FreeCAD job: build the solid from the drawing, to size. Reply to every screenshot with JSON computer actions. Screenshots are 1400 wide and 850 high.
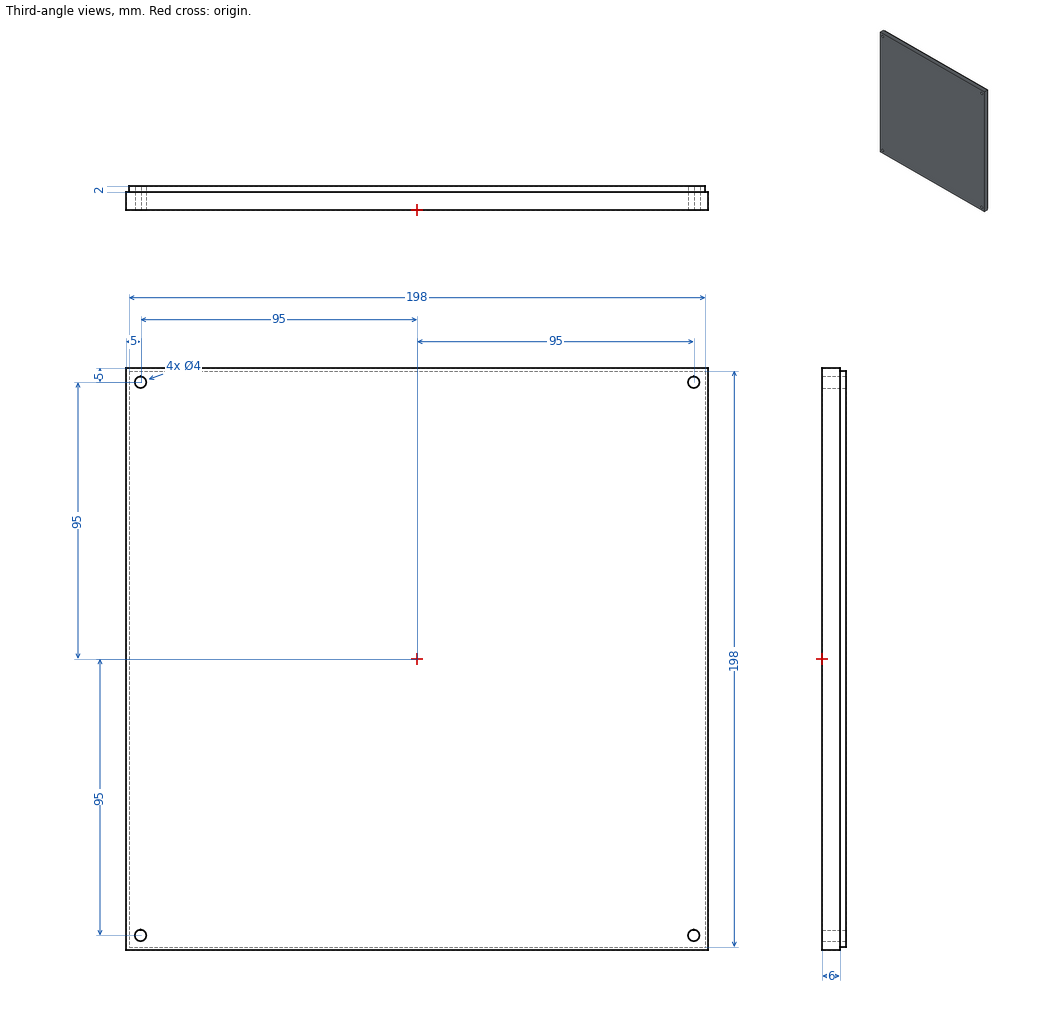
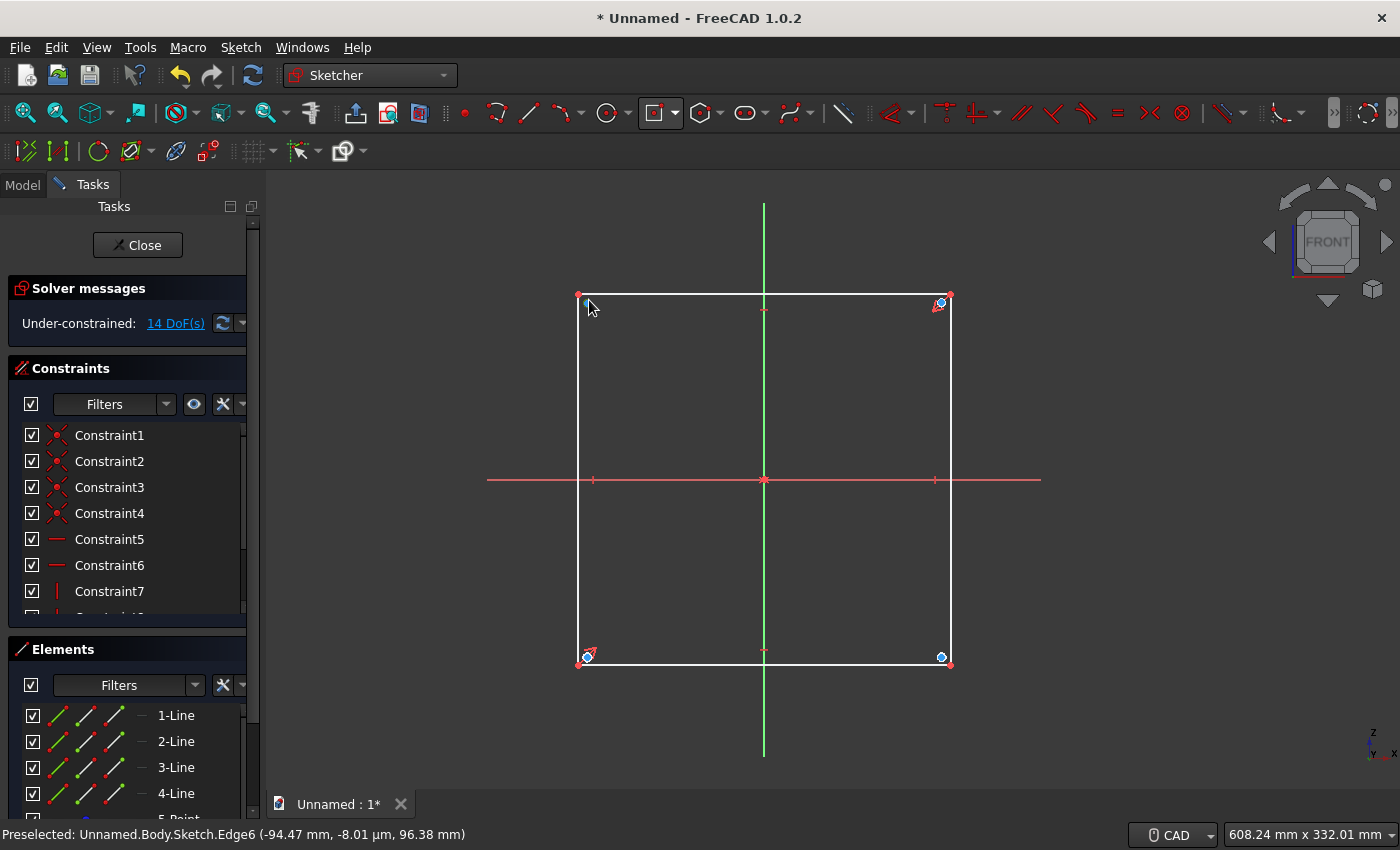
{"action": "scroll", "coordinate": [944, 300], "scroll_direction": "up", "scroll_amount": 7}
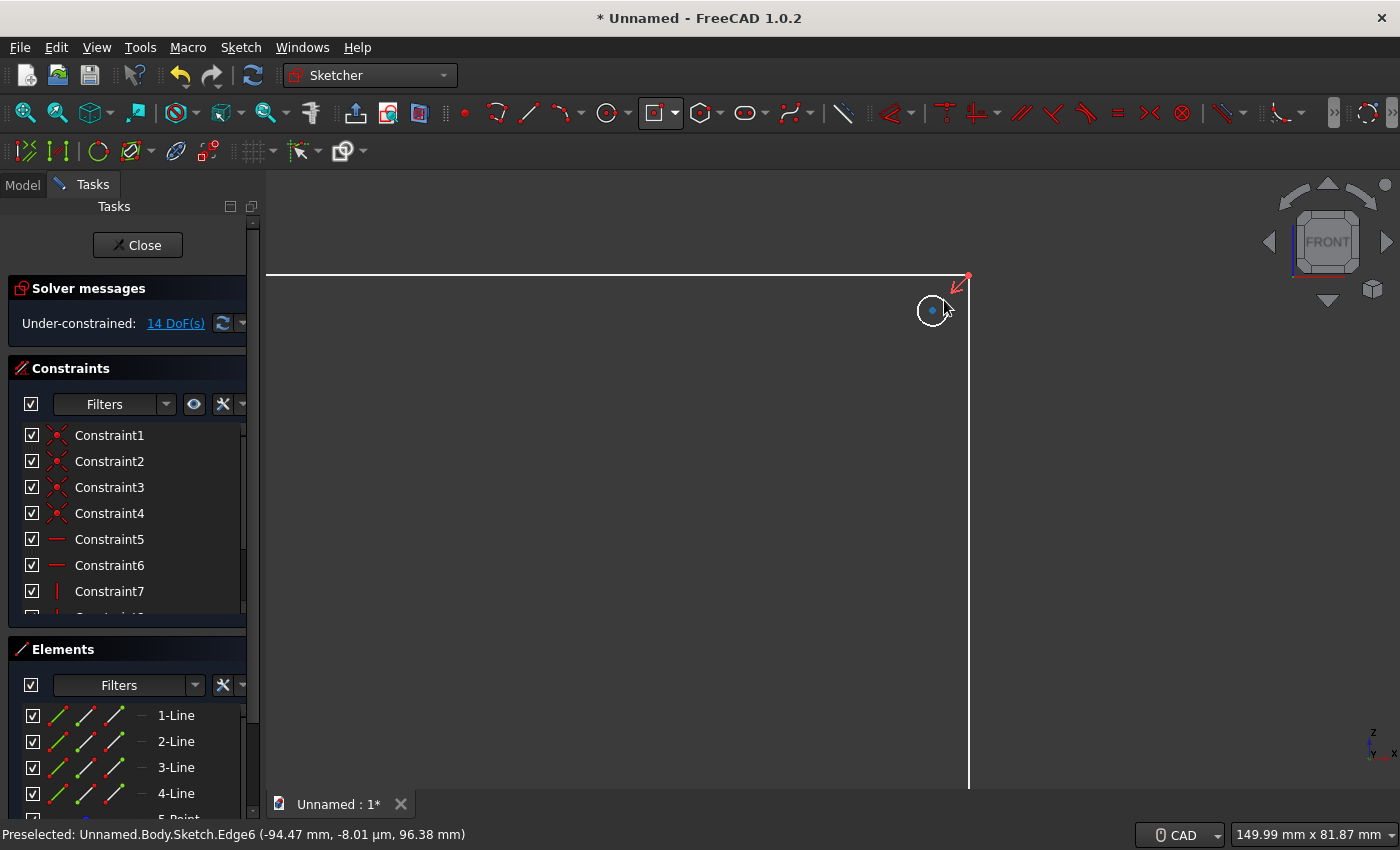
{"action": "left_click", "coordinate": [943, 300]}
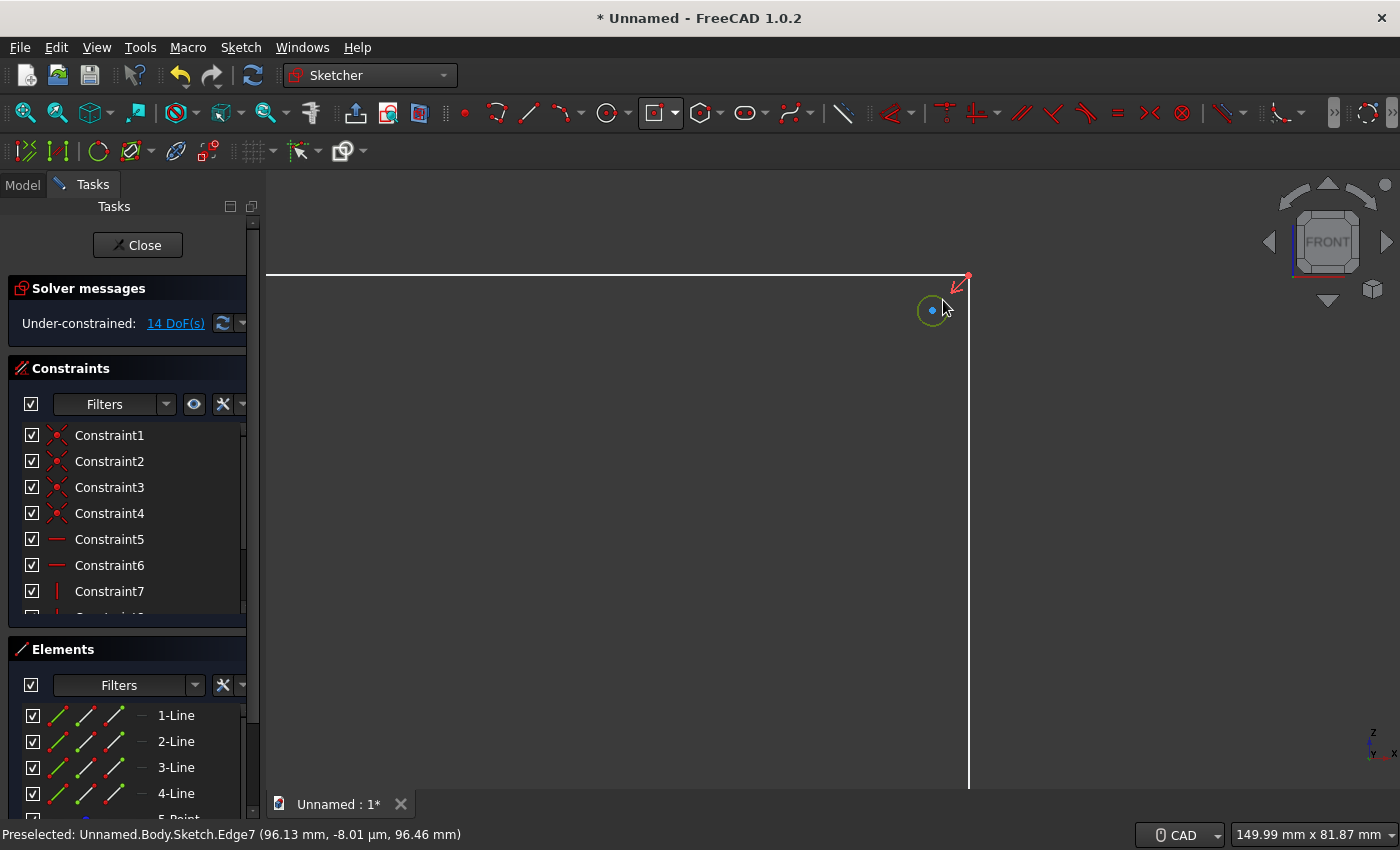
{"action": "scroll", "coordinate": [945, 300], "scroll_direction": "down", "scroll_amount": 7}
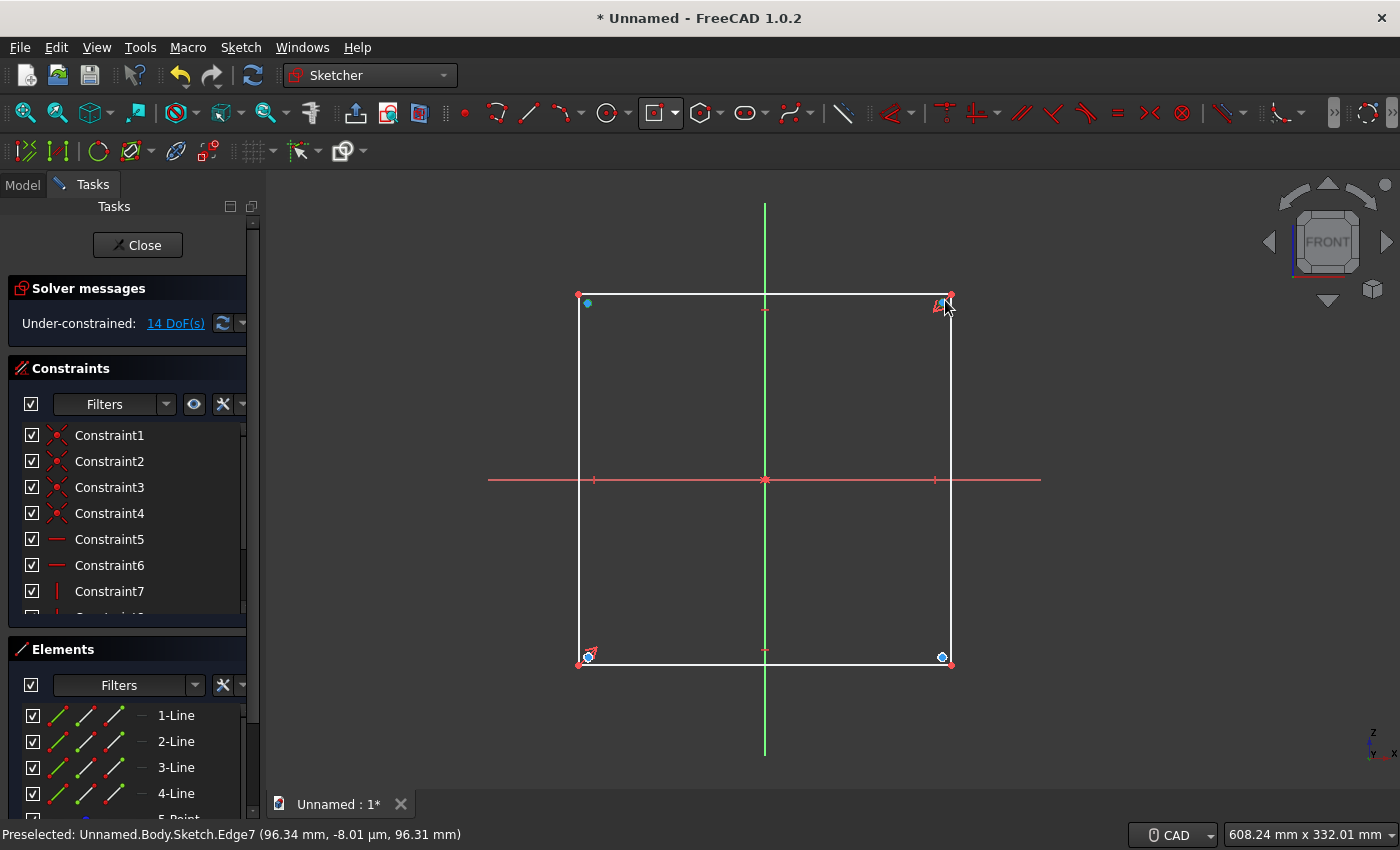
{"action": "scroll", "coordinate": [591, 654], "scroll_direction": "up", "scroll_amount": 6}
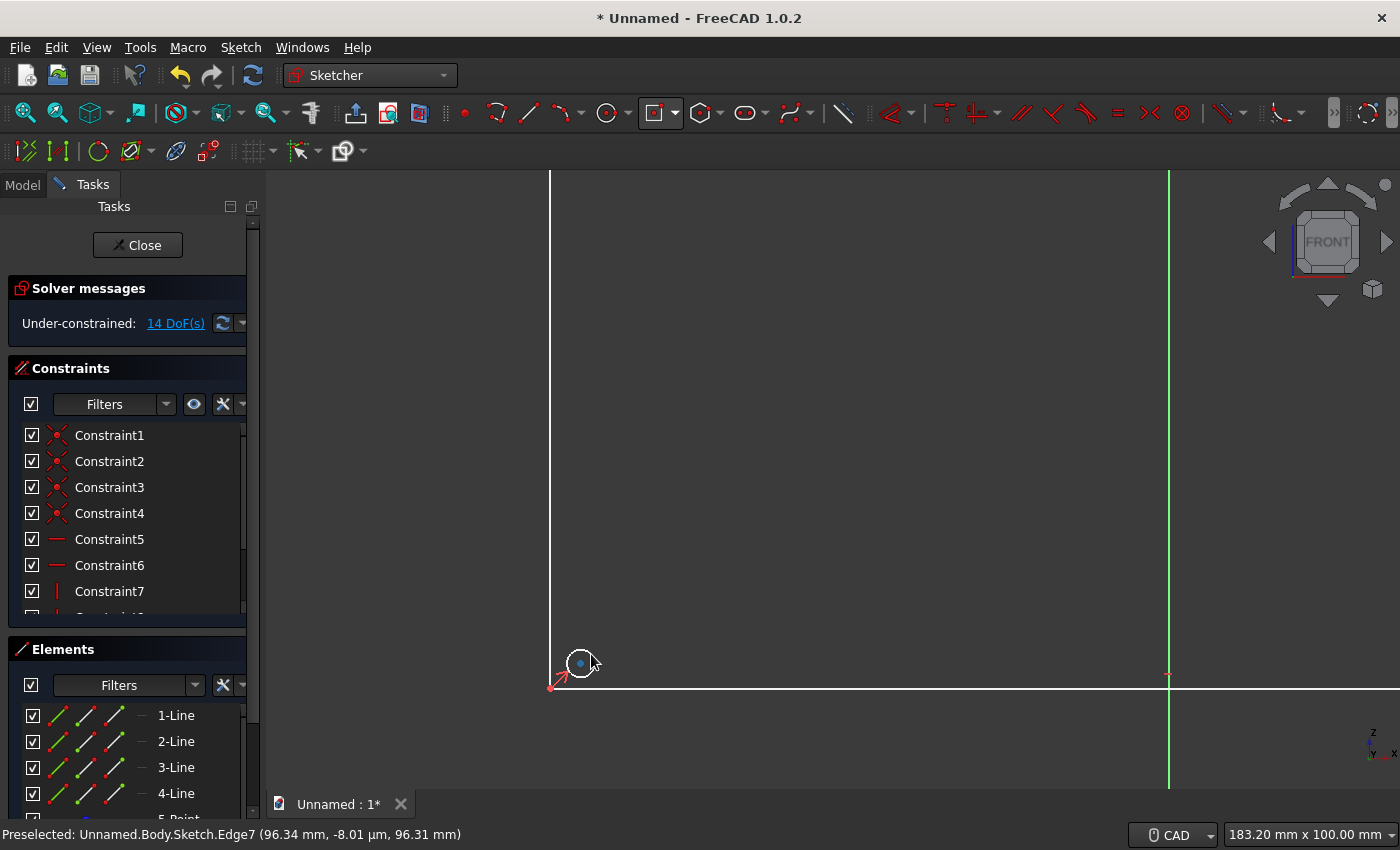
{"action": "left_click", "coordinate": [591, 654]}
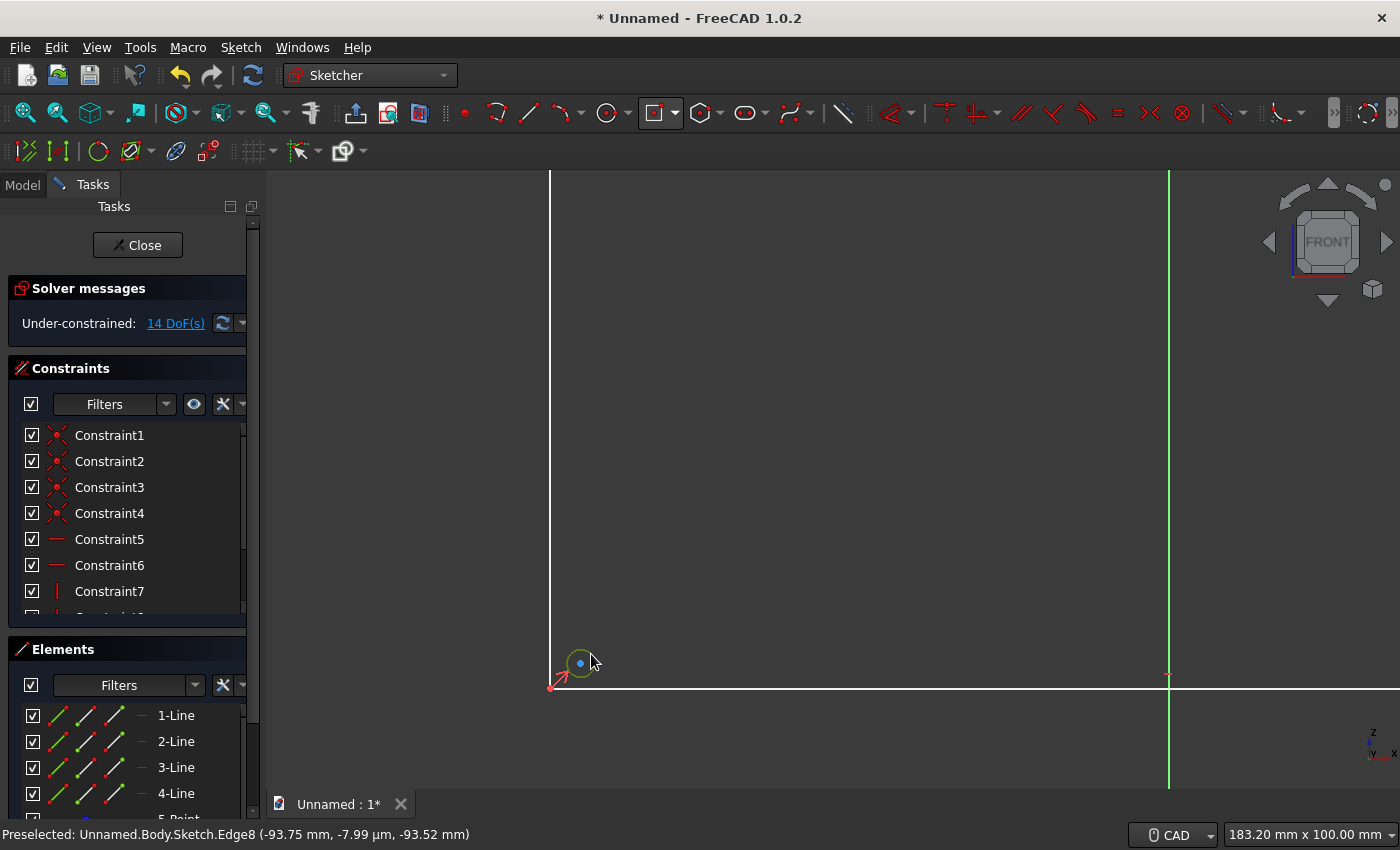
{"action": "scroll", "coordinate": [590, 655], "scroll_direction": "down", "scroll_amount": 6}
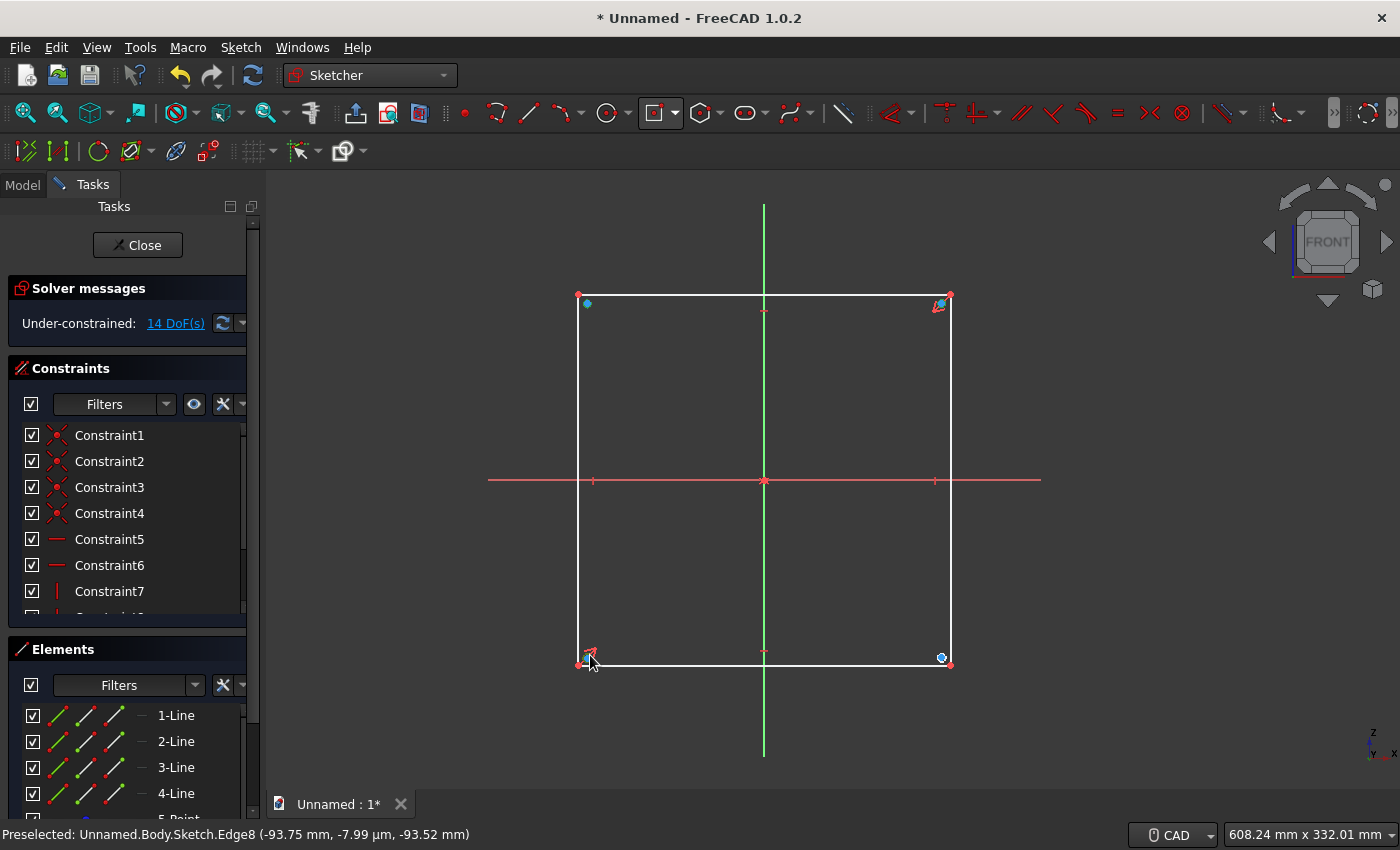
{"action": "scroll", "coordinate": [945, 655], "scroll_direction": "up", "scroll_amount": 7}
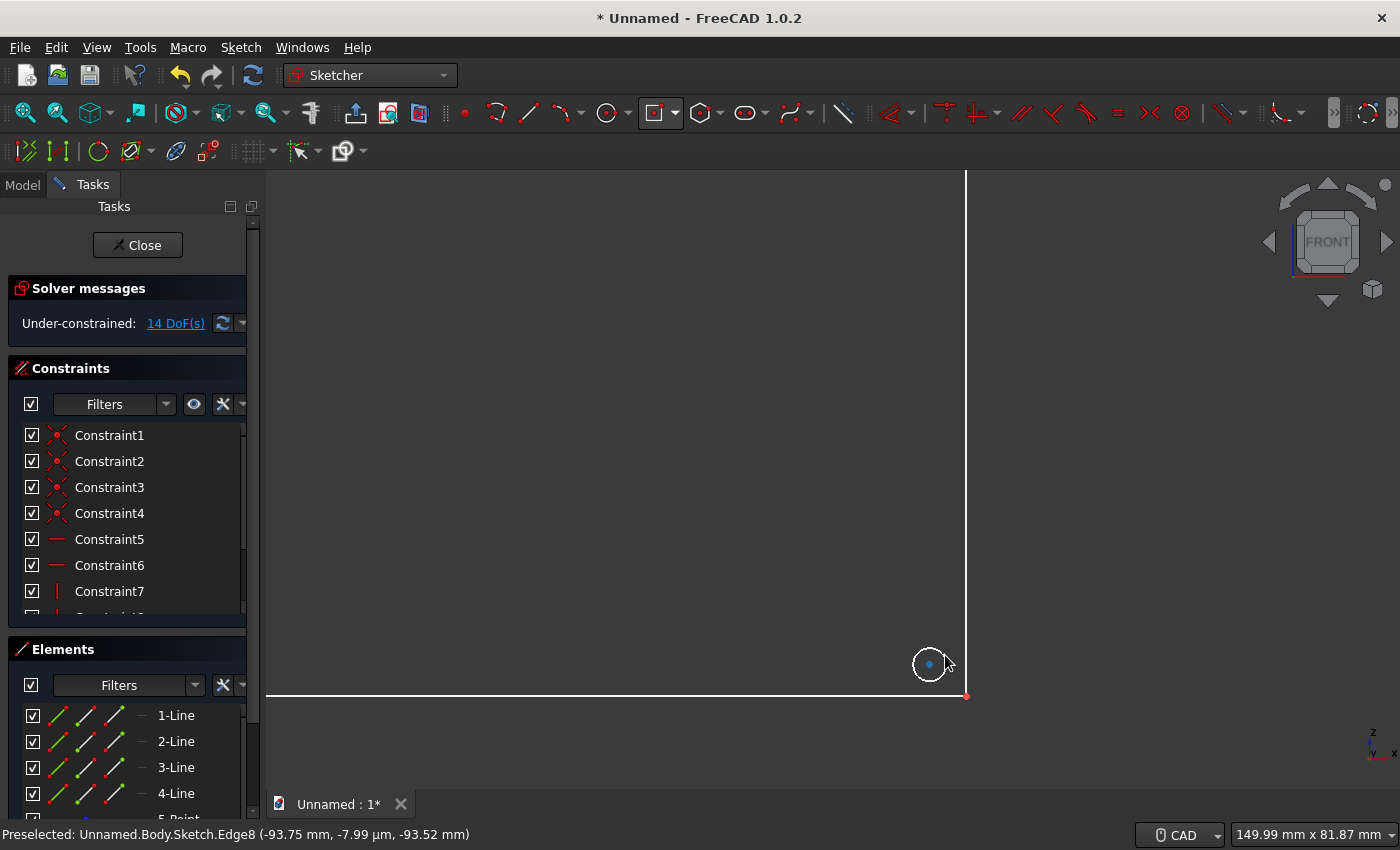
{"action": "left_click", "coordinate": [941, 653]}